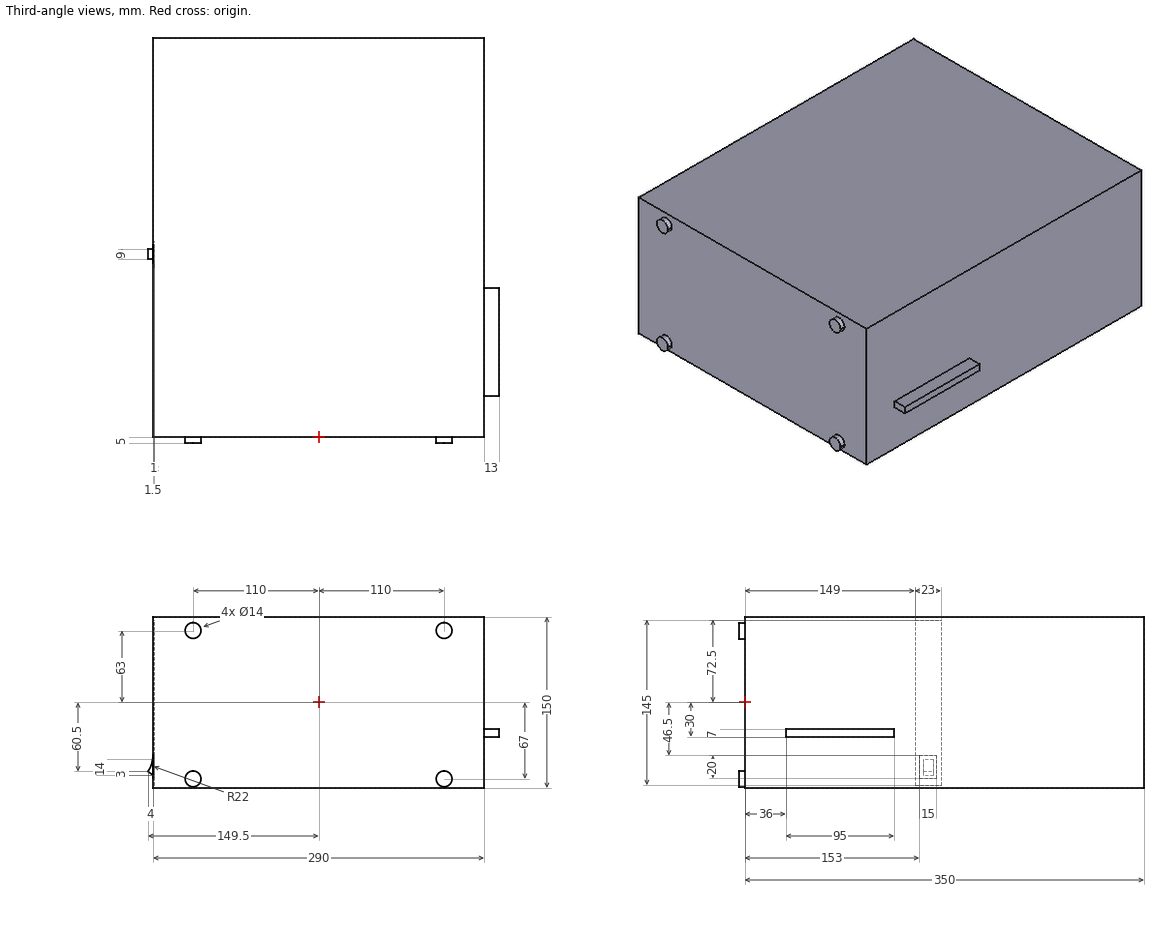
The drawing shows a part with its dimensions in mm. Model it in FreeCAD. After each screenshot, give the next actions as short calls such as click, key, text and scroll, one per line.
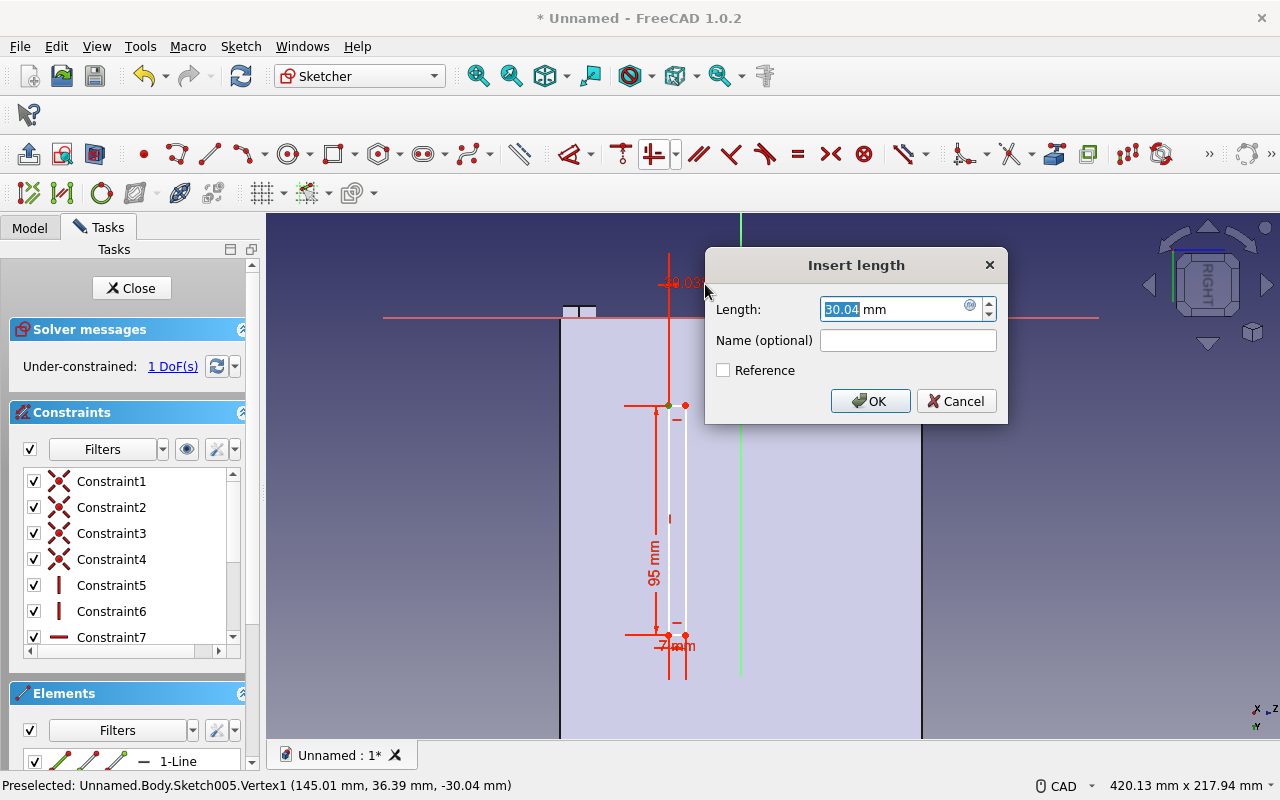
text(30)
key(Return)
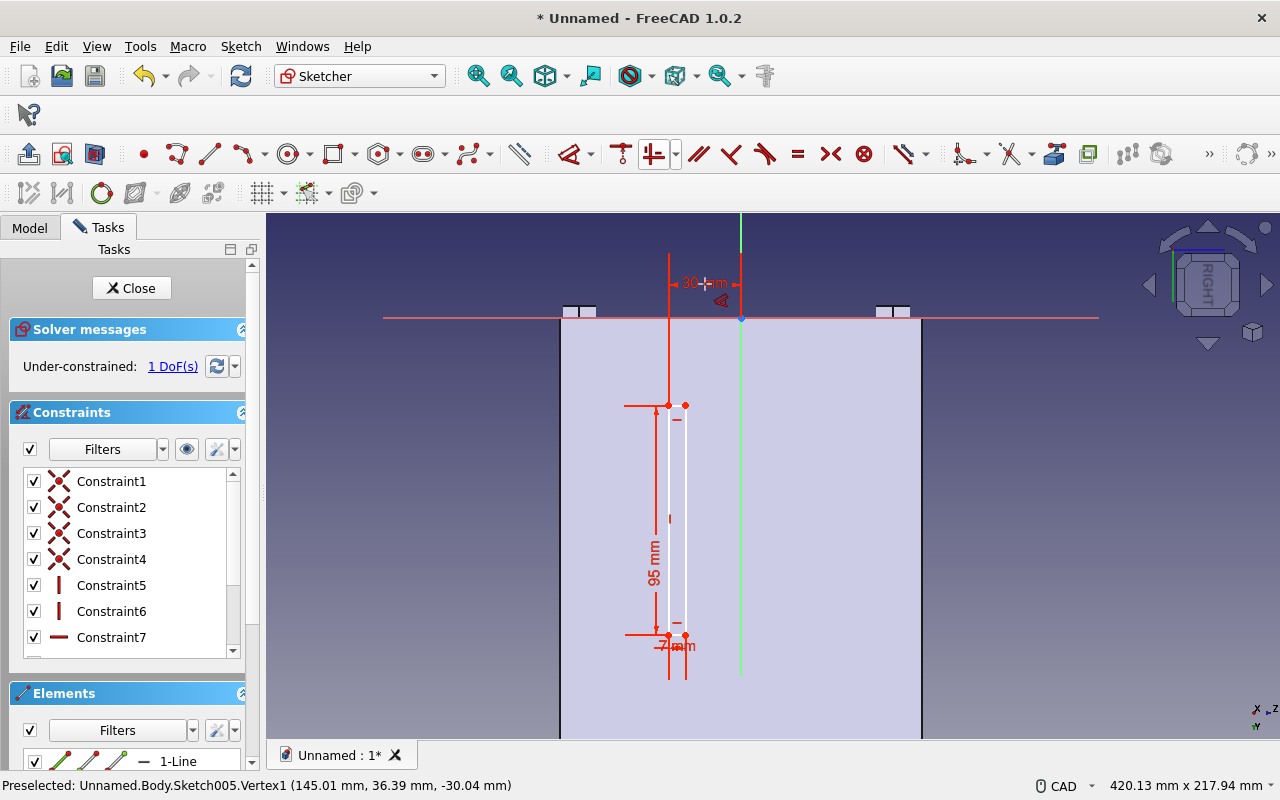
click(669, 406)
click(775, 362)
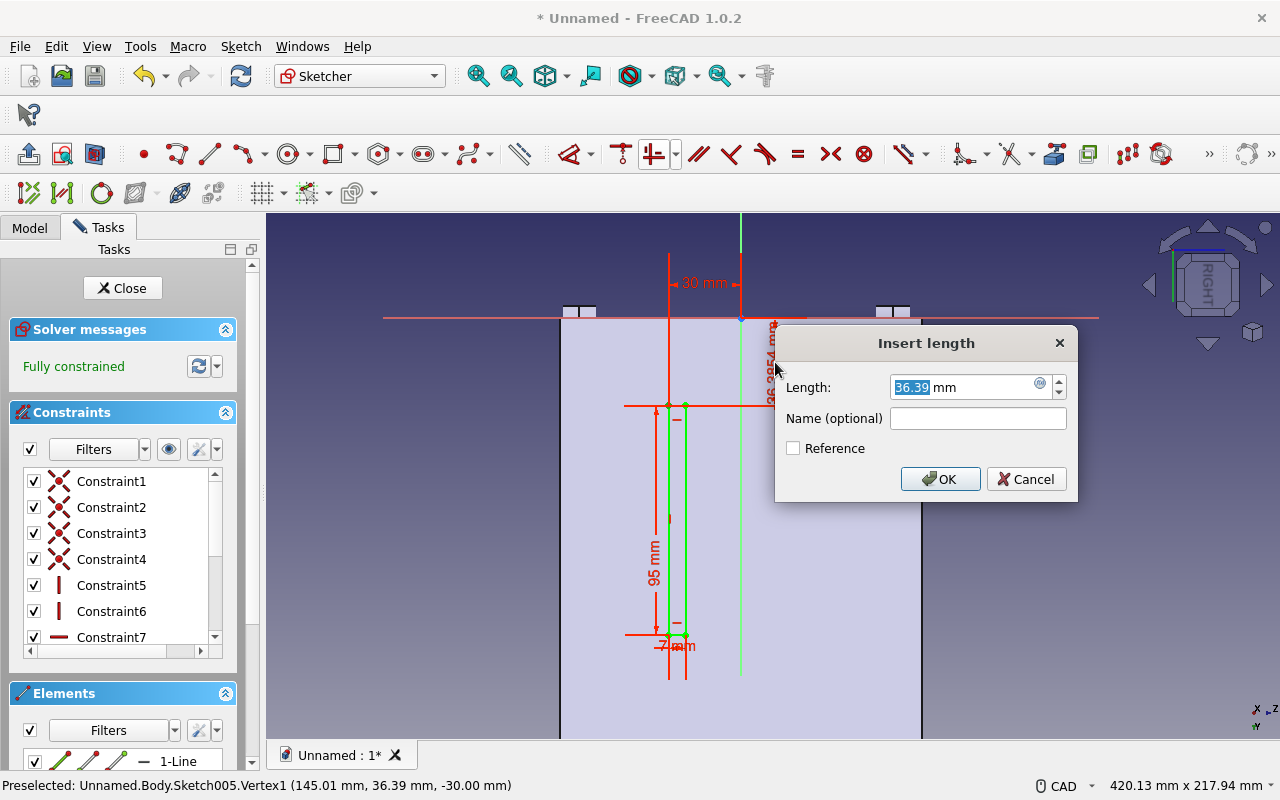
text(36)
key(Return)
key(Escape)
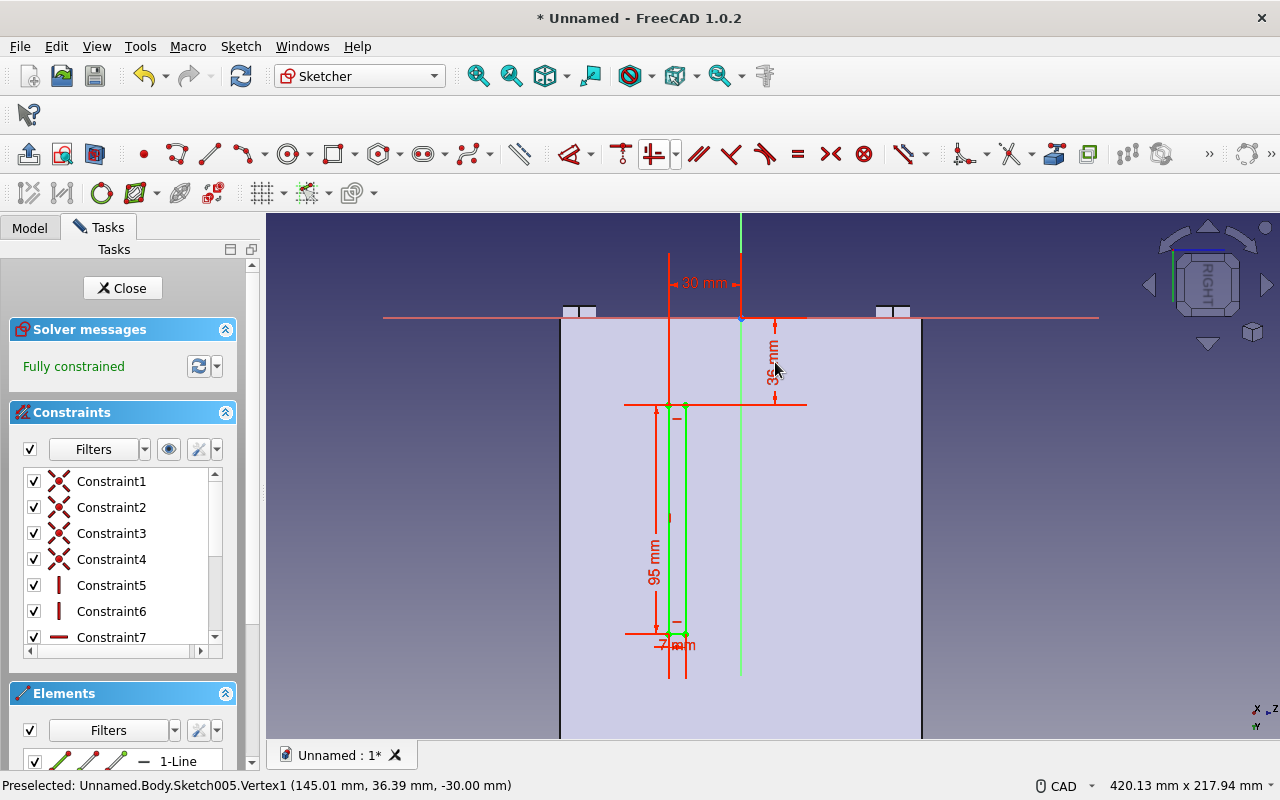
click(123, 288)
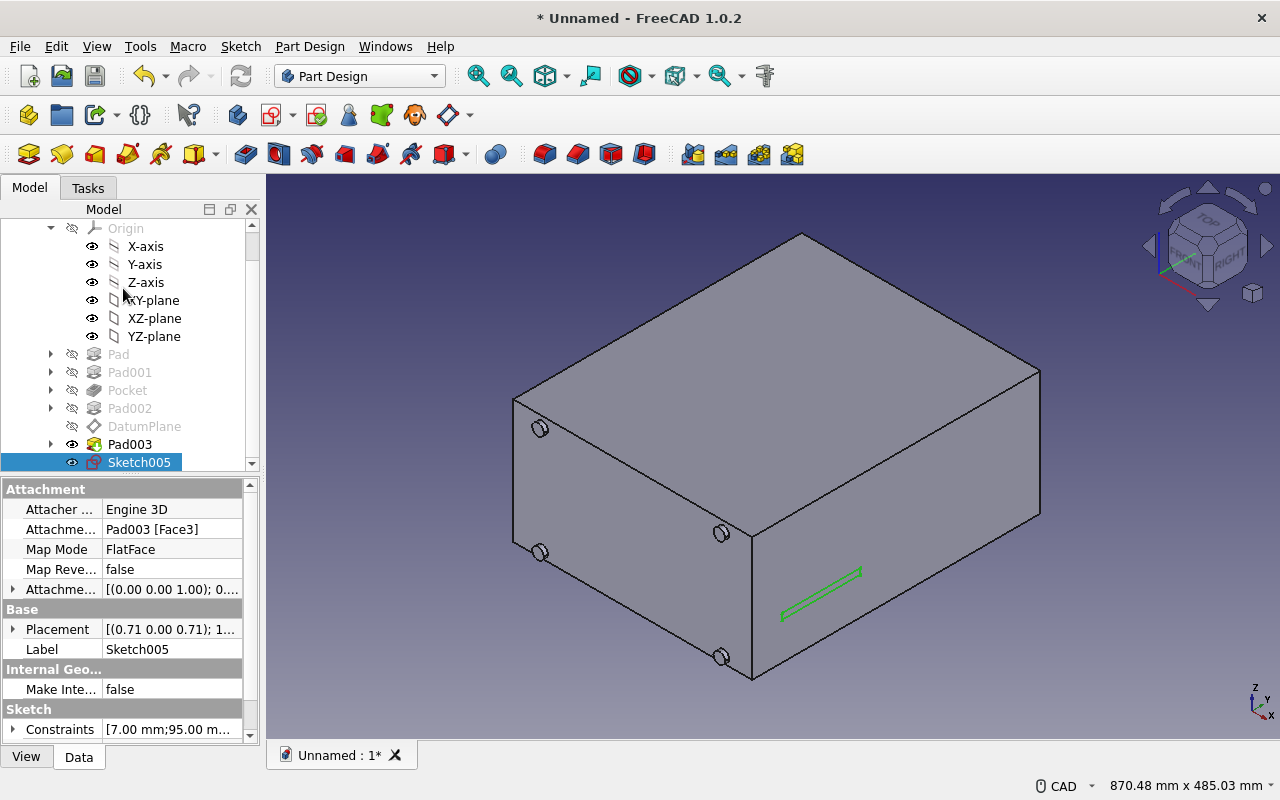
click(29, 154)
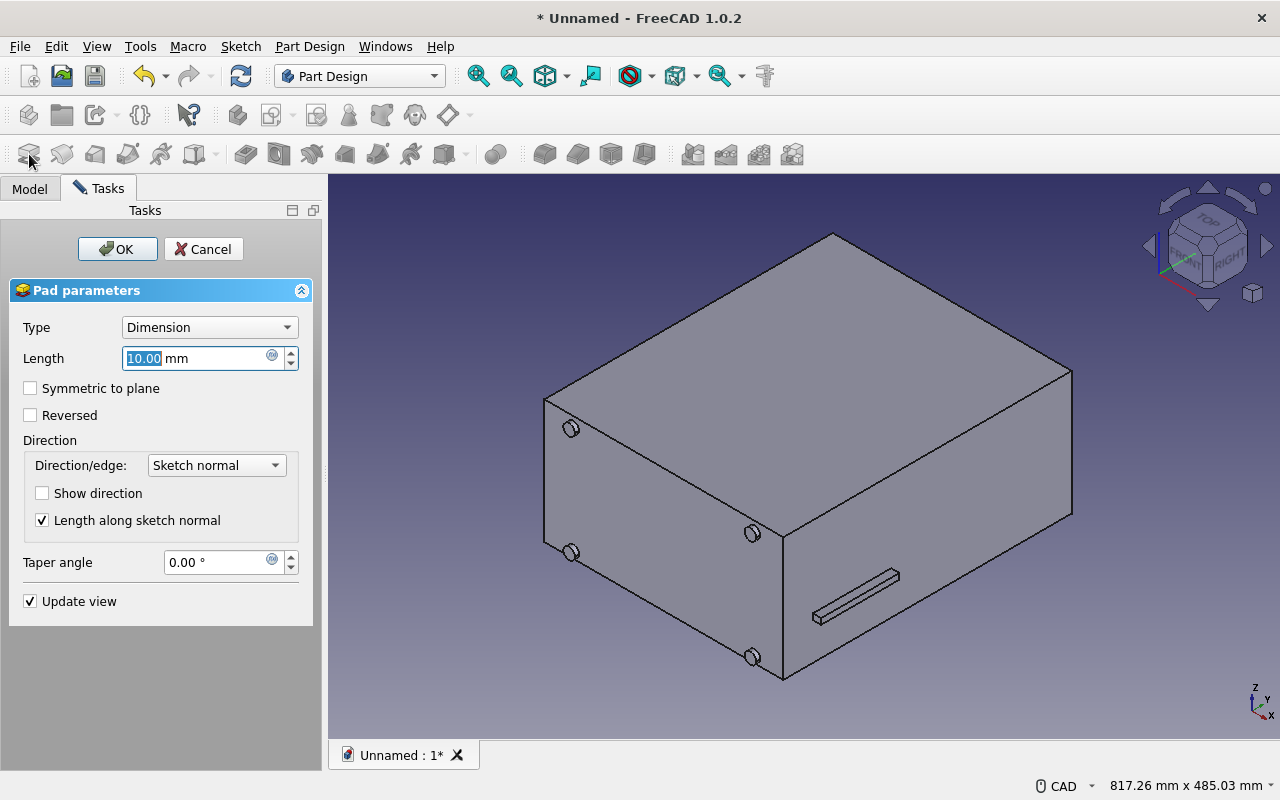
text(13)
key(Tab)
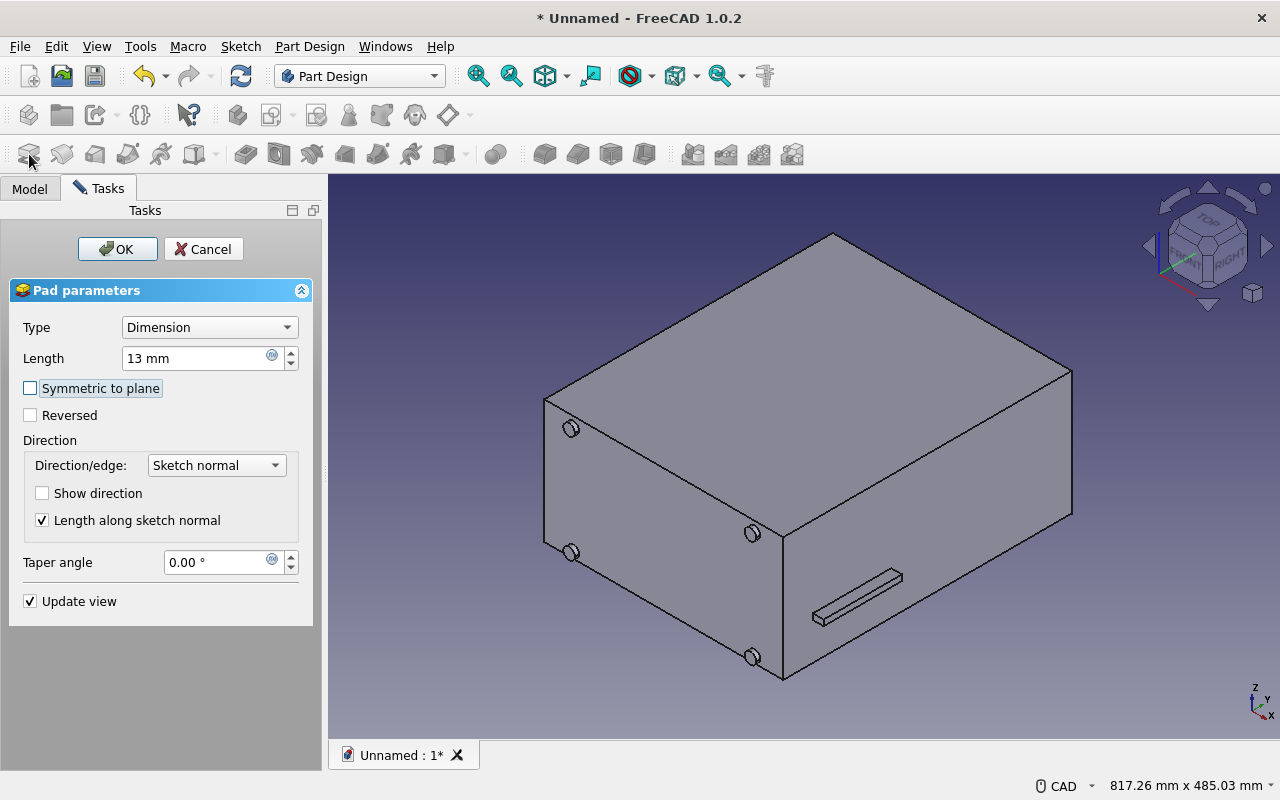
click(118, 249)